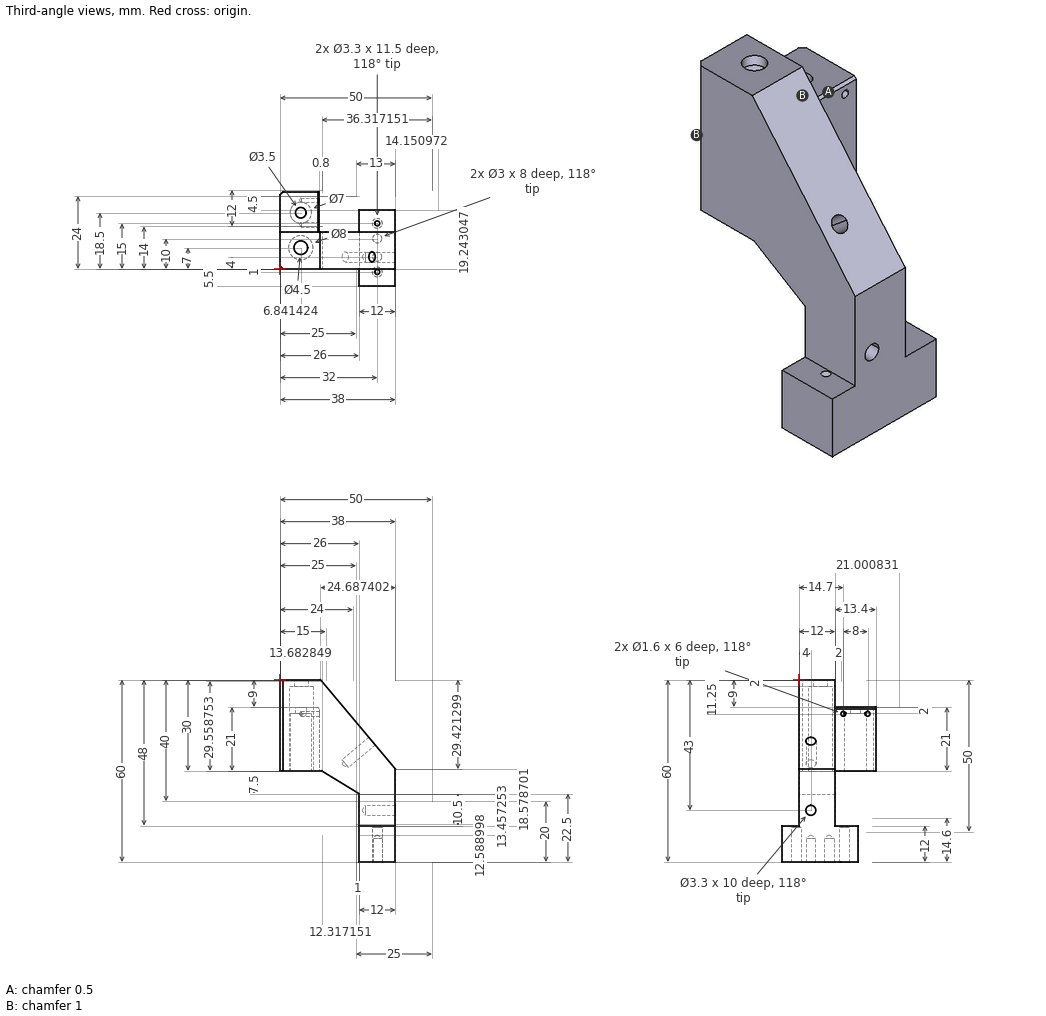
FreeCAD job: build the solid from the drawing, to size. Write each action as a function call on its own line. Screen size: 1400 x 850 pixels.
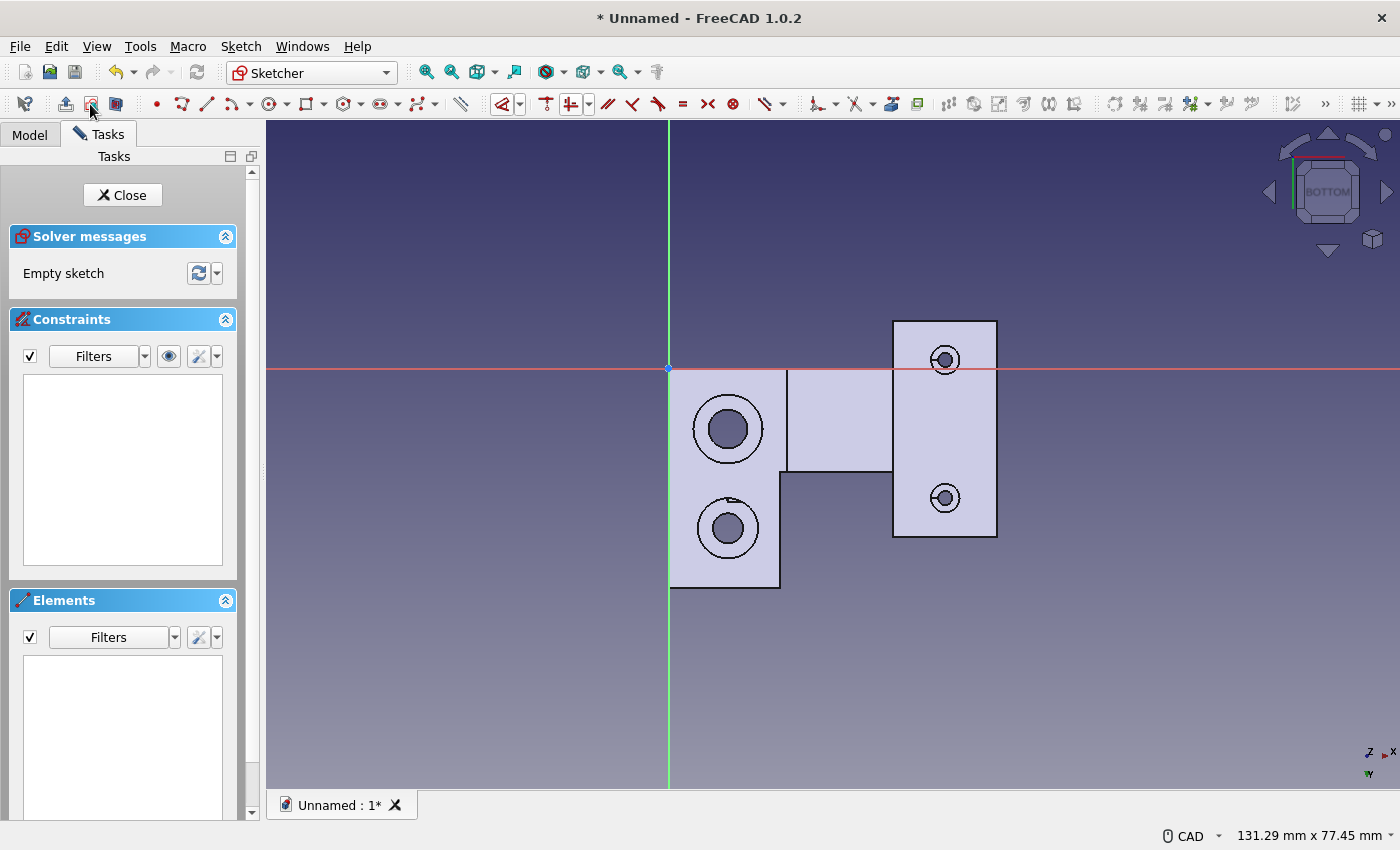
scroll(981, 424, up, 9)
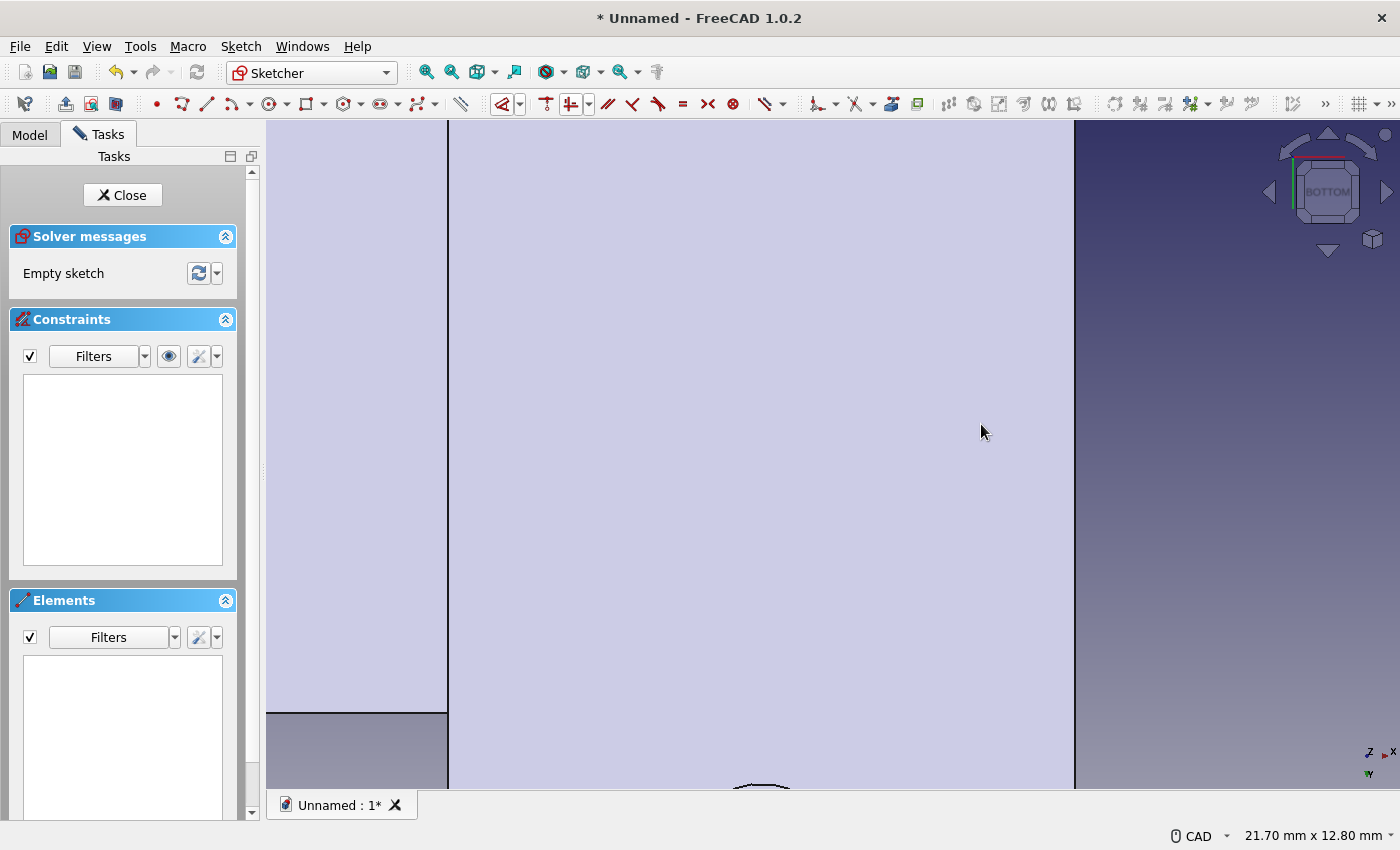
click(268, 104)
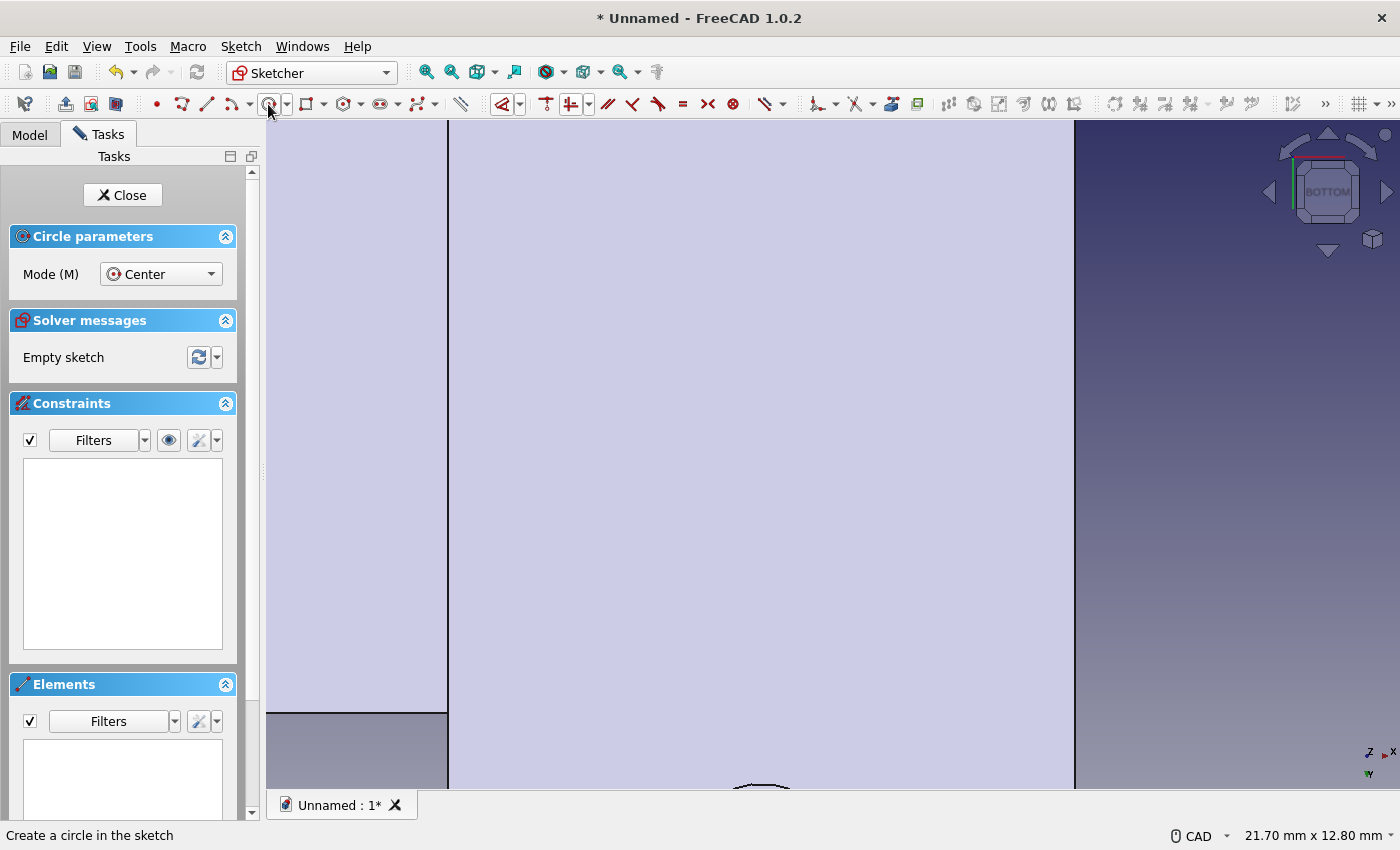
click(762, 609)
click(817, 553)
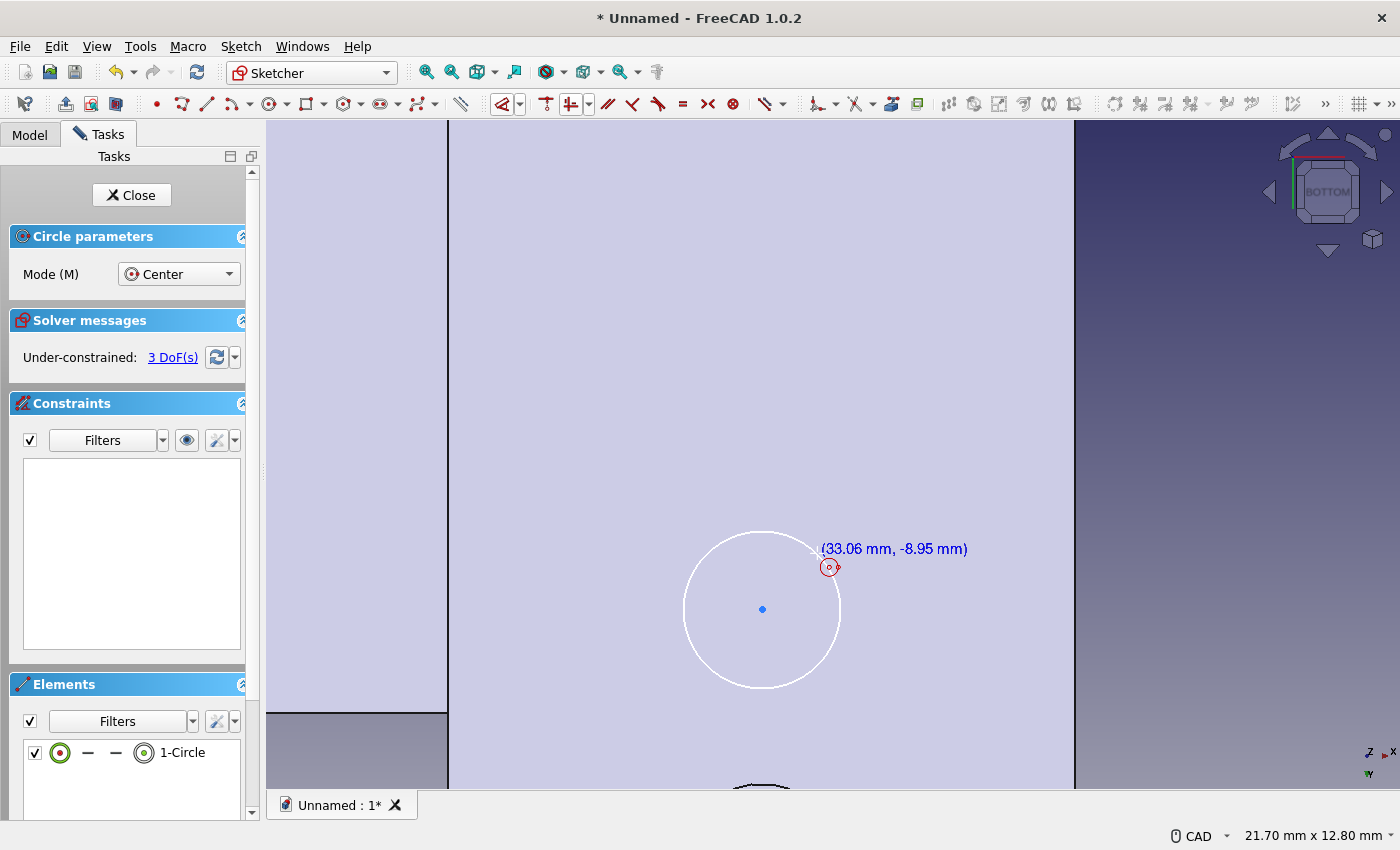
click(762, 295)
click(817, 240)
key(Escape)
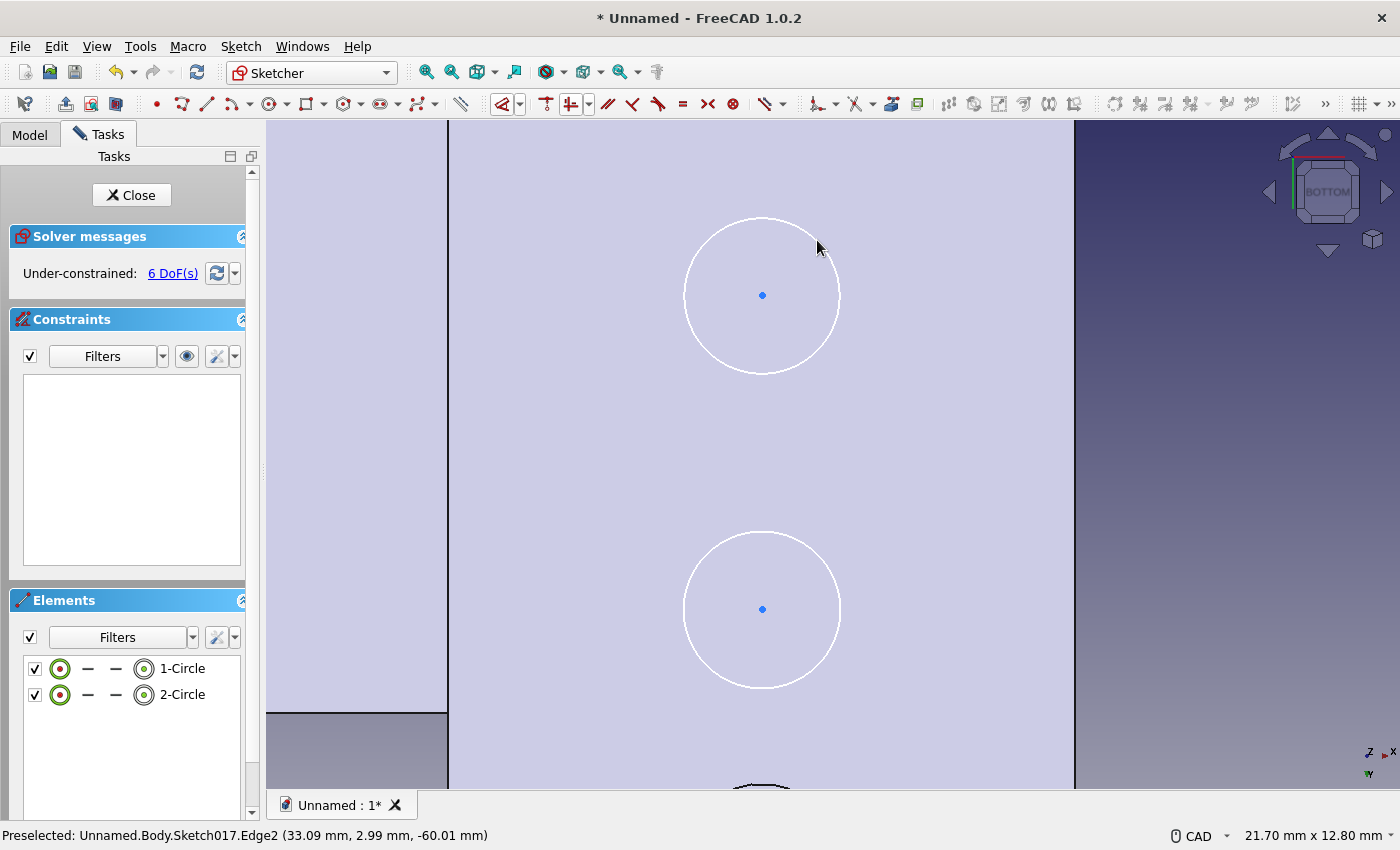
click(817, 554)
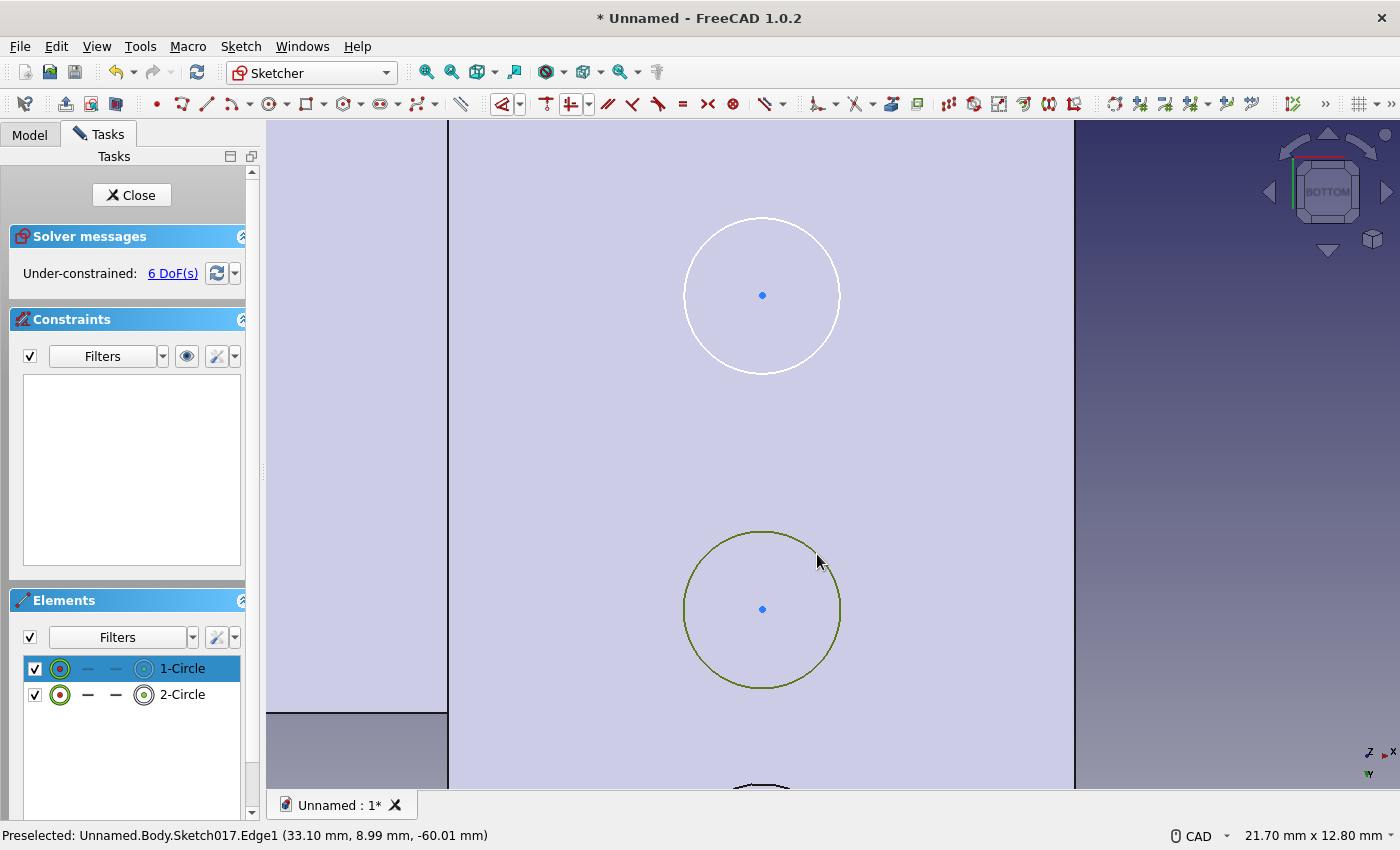
click(817, 241)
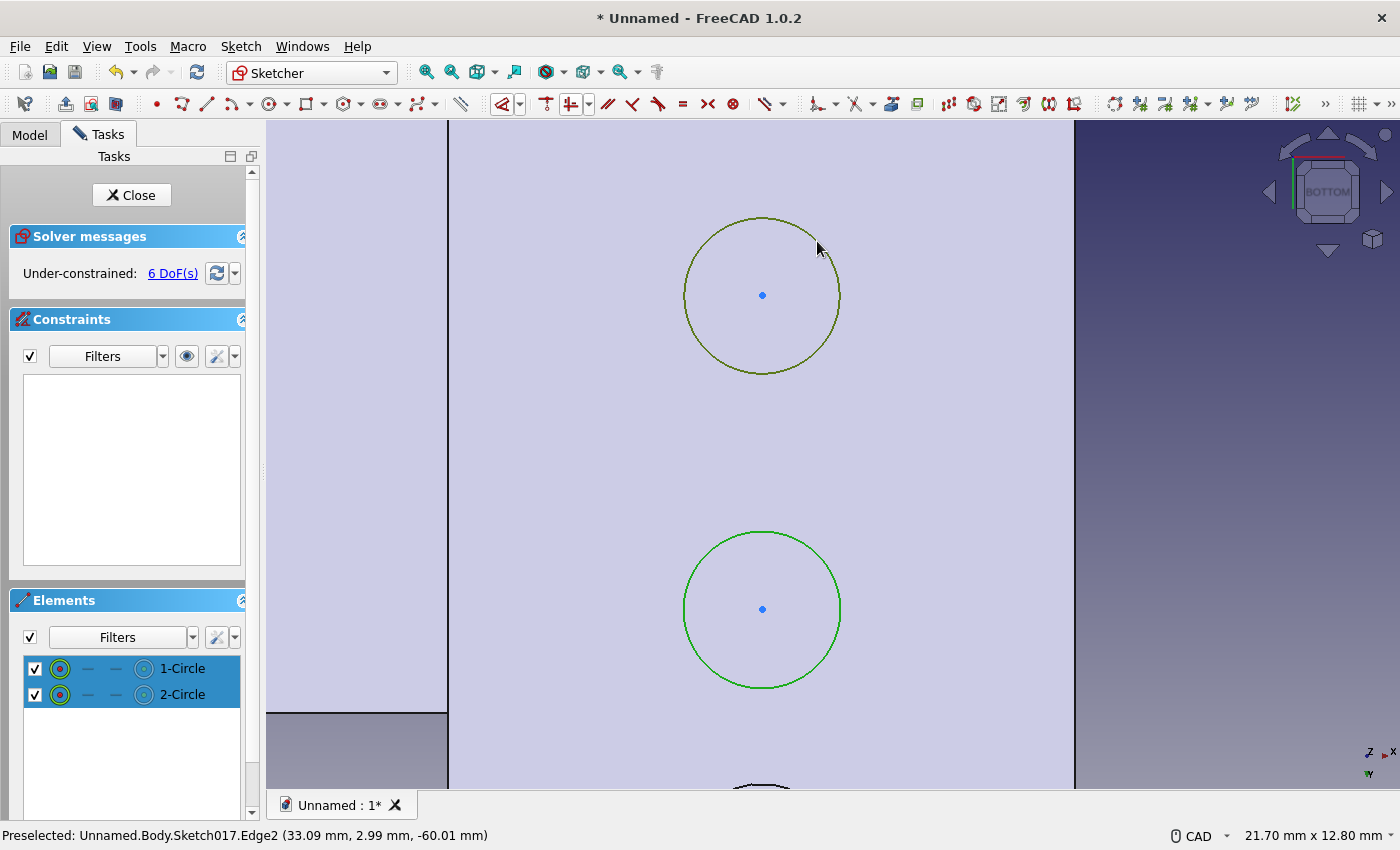
click(683, 104)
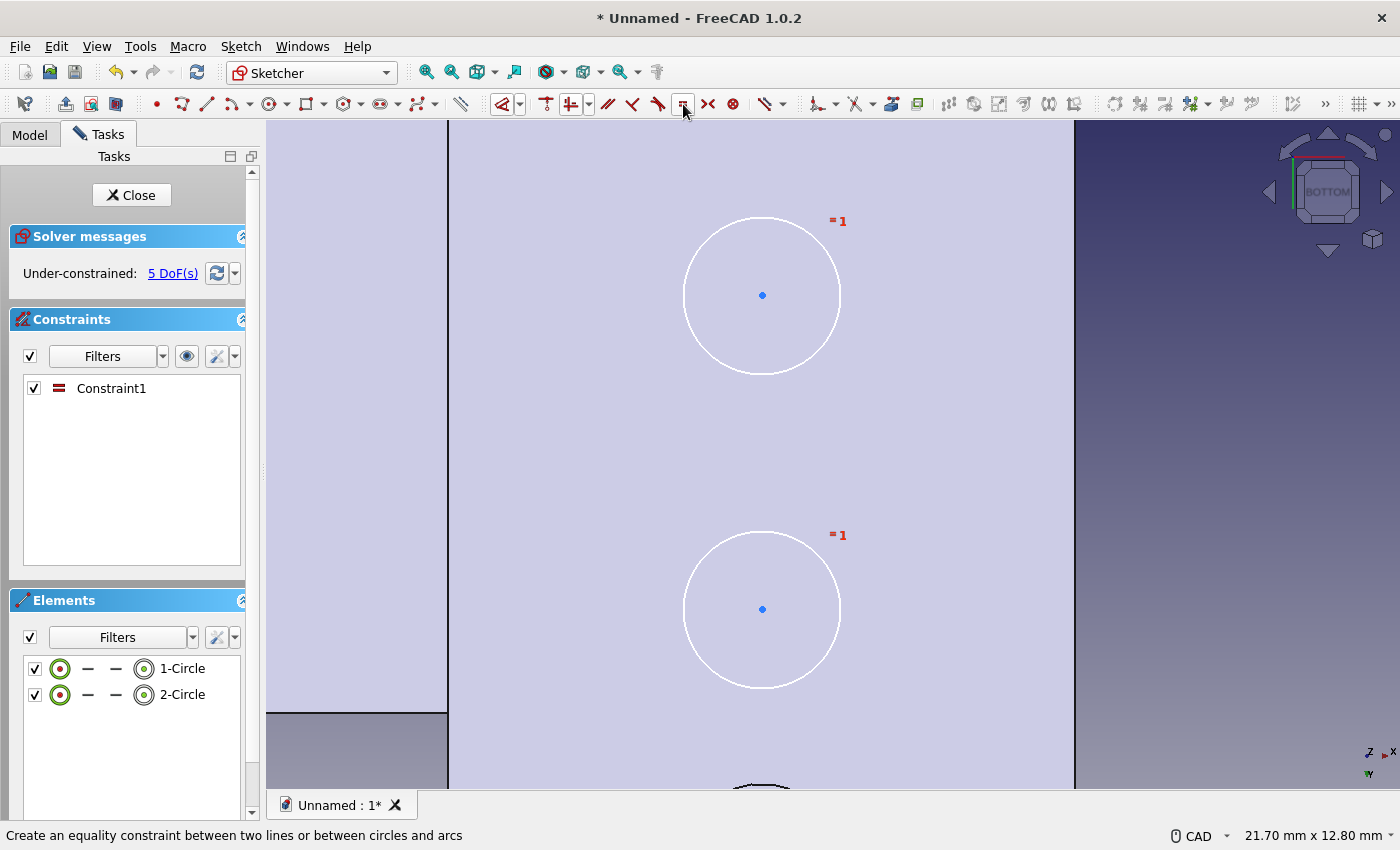
click(762, 610)